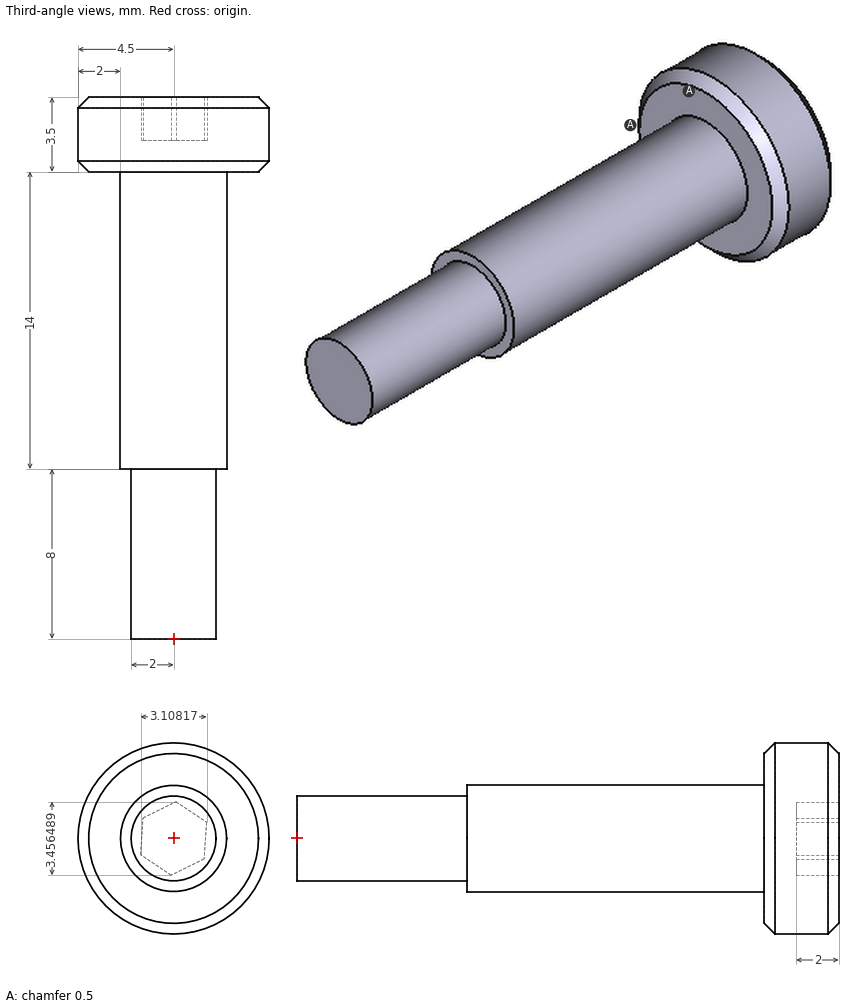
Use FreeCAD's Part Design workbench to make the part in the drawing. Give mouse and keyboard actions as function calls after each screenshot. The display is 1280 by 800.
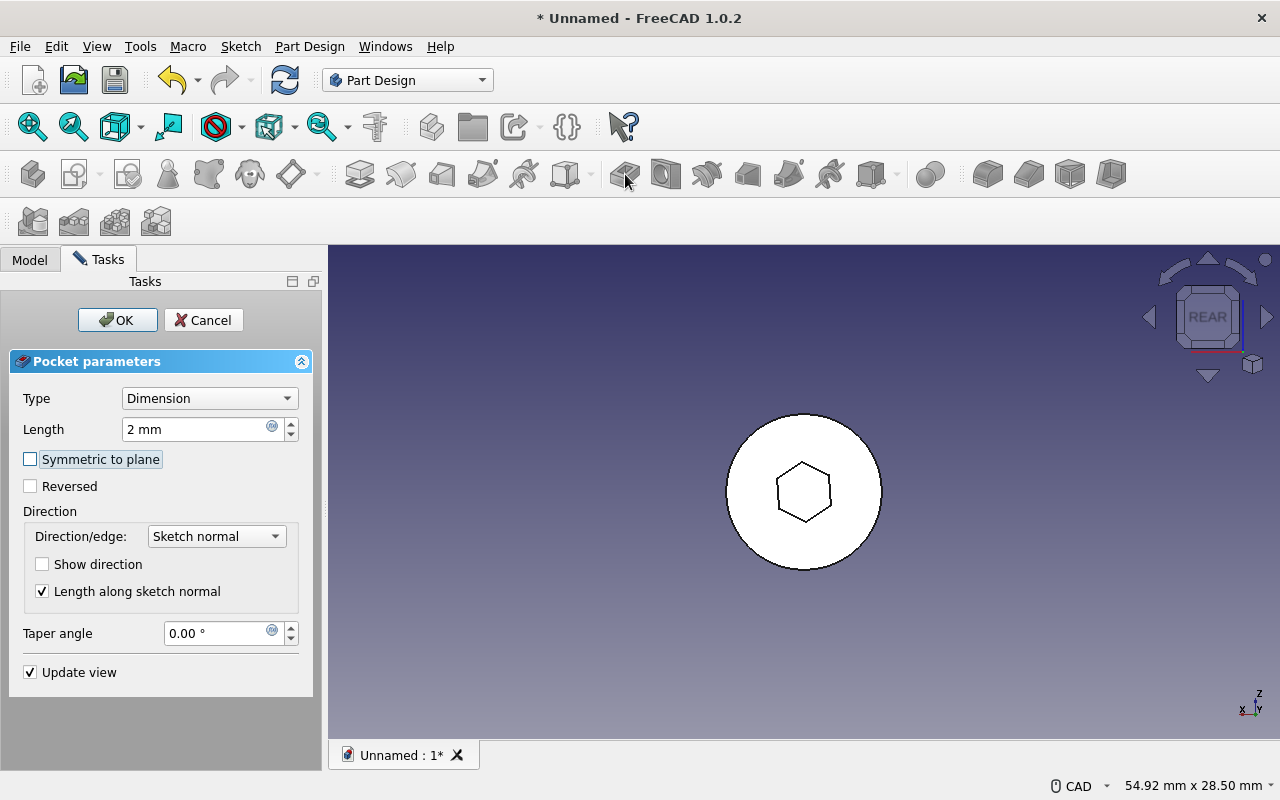
click(118, 320)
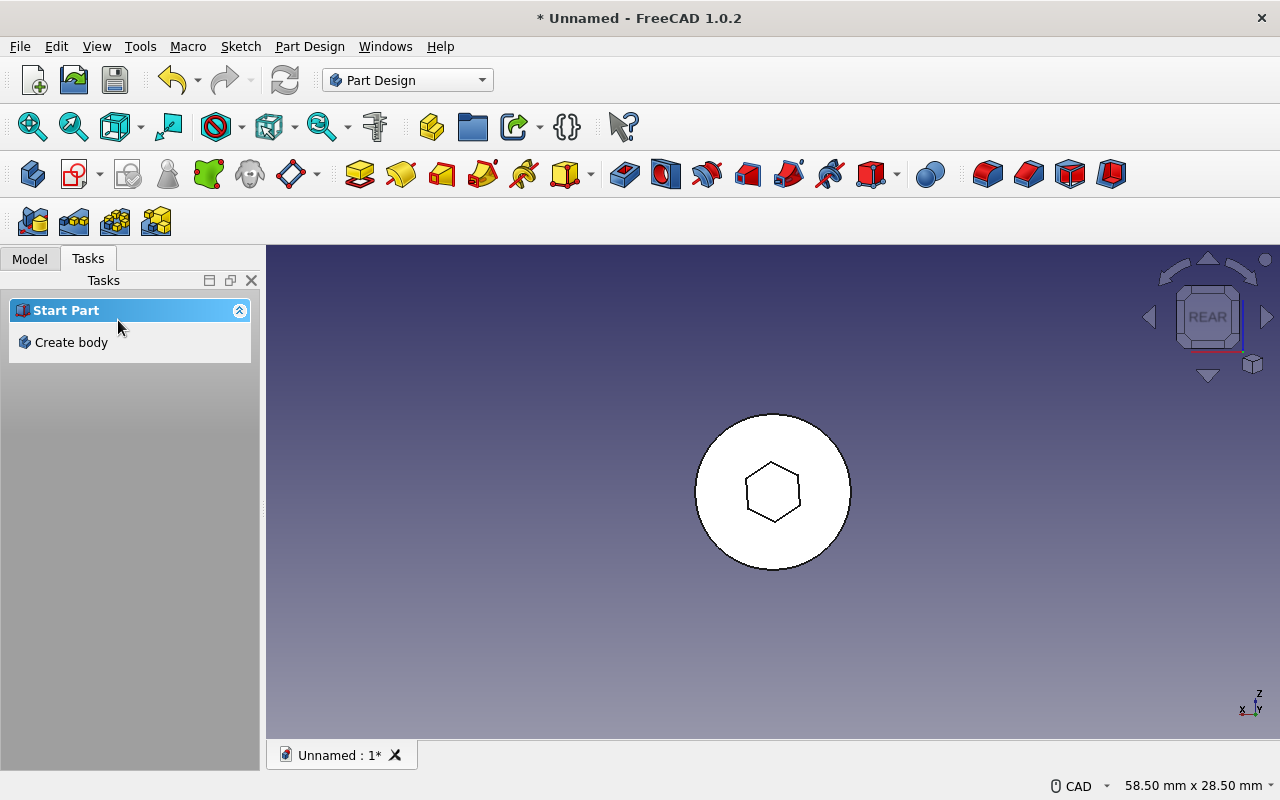
click(33, 128)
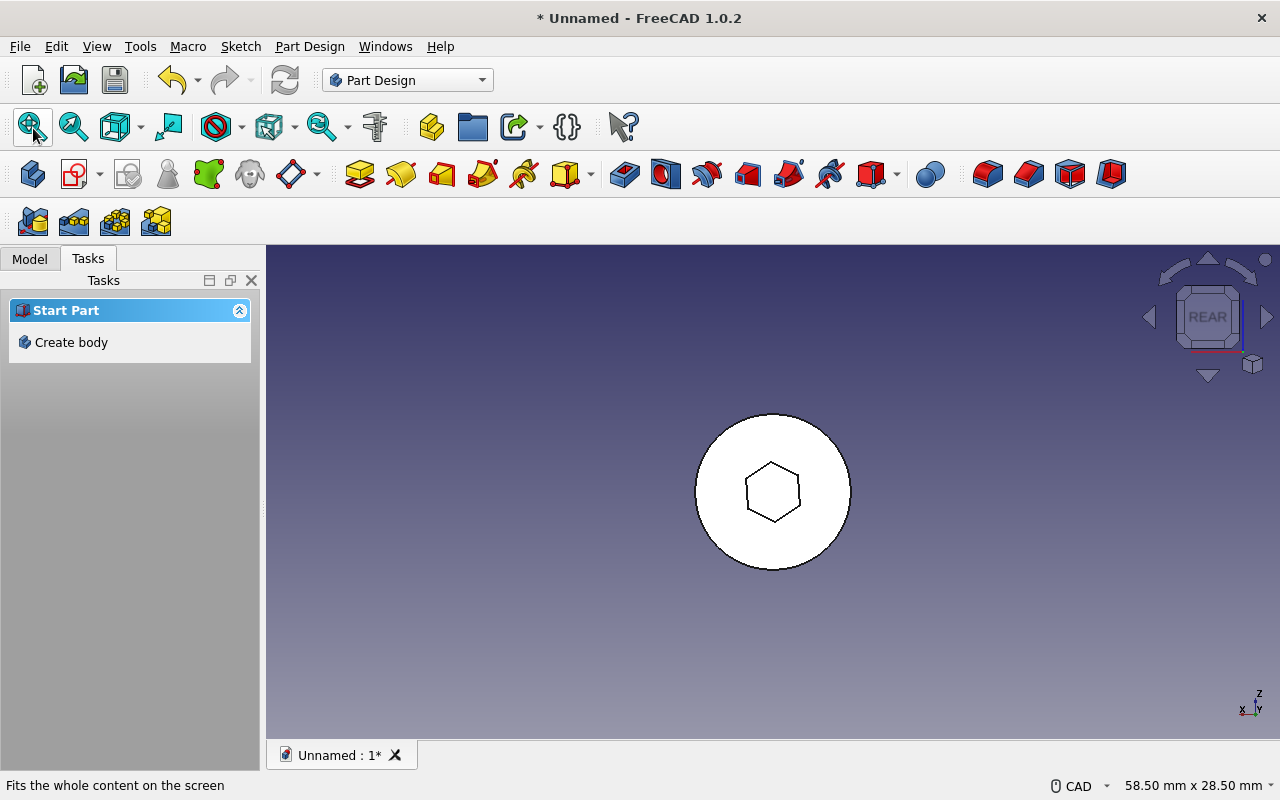
click(797, 417)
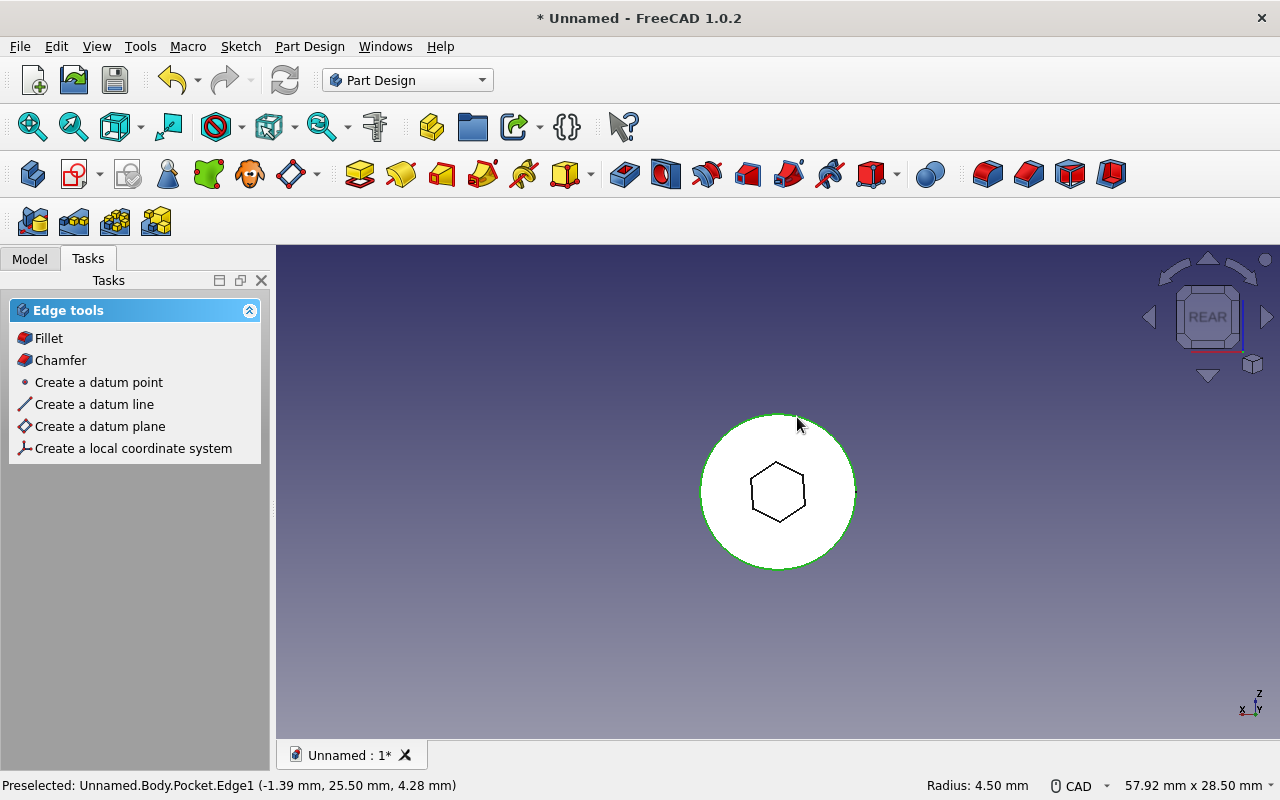
key(0)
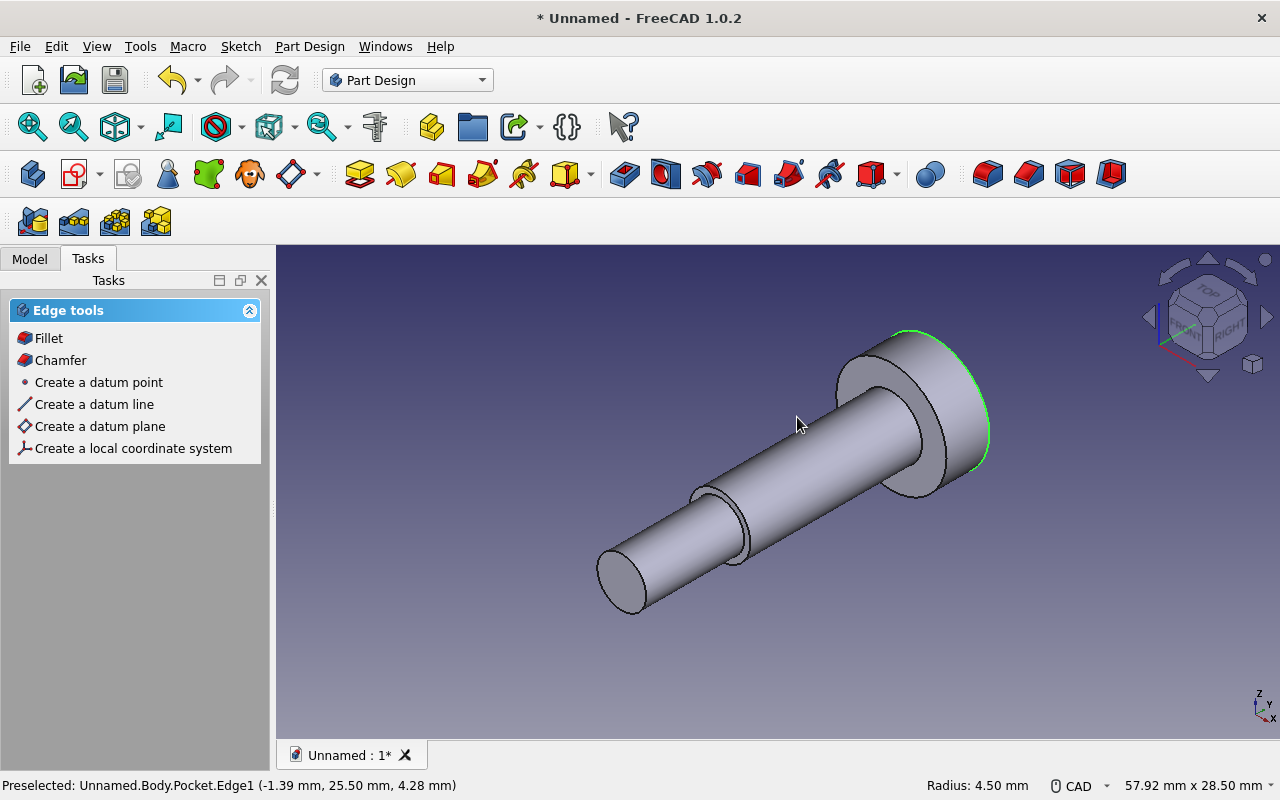
click(947, 457, ctrl)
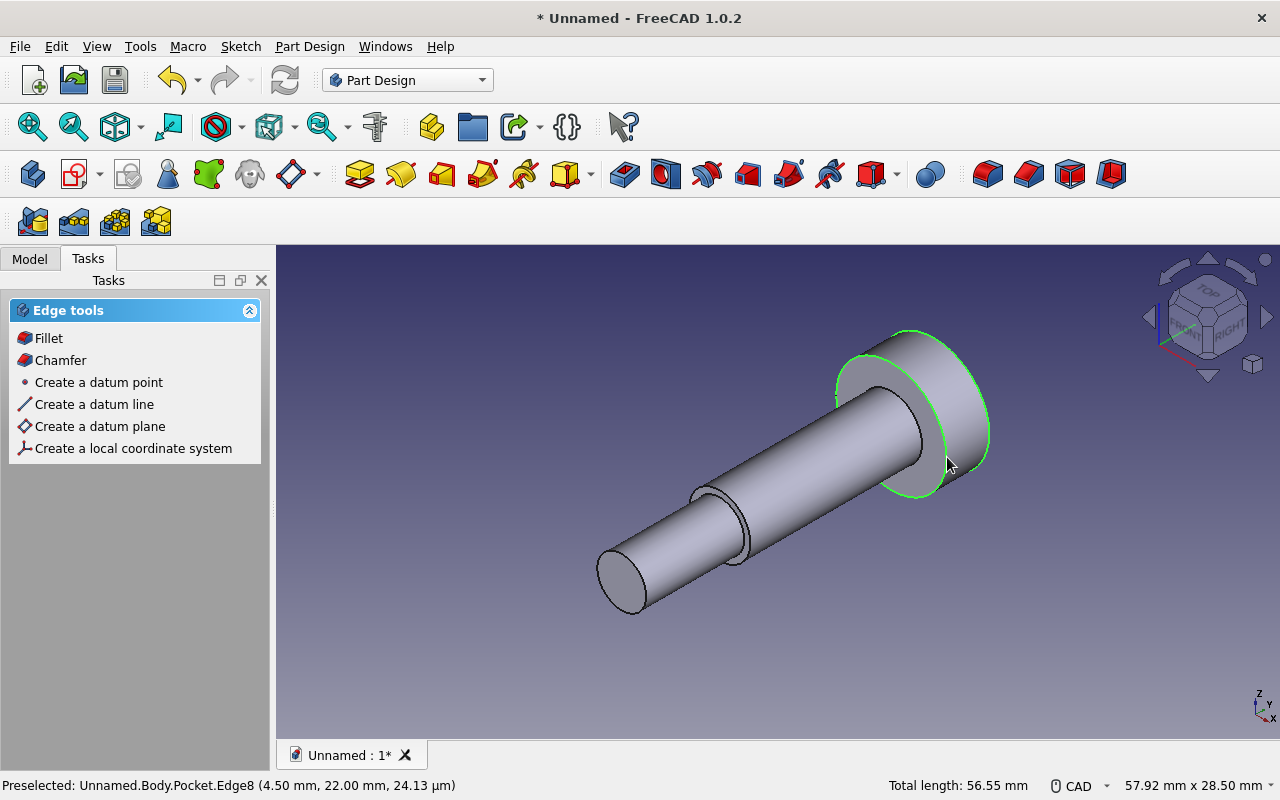
click(1029, 174)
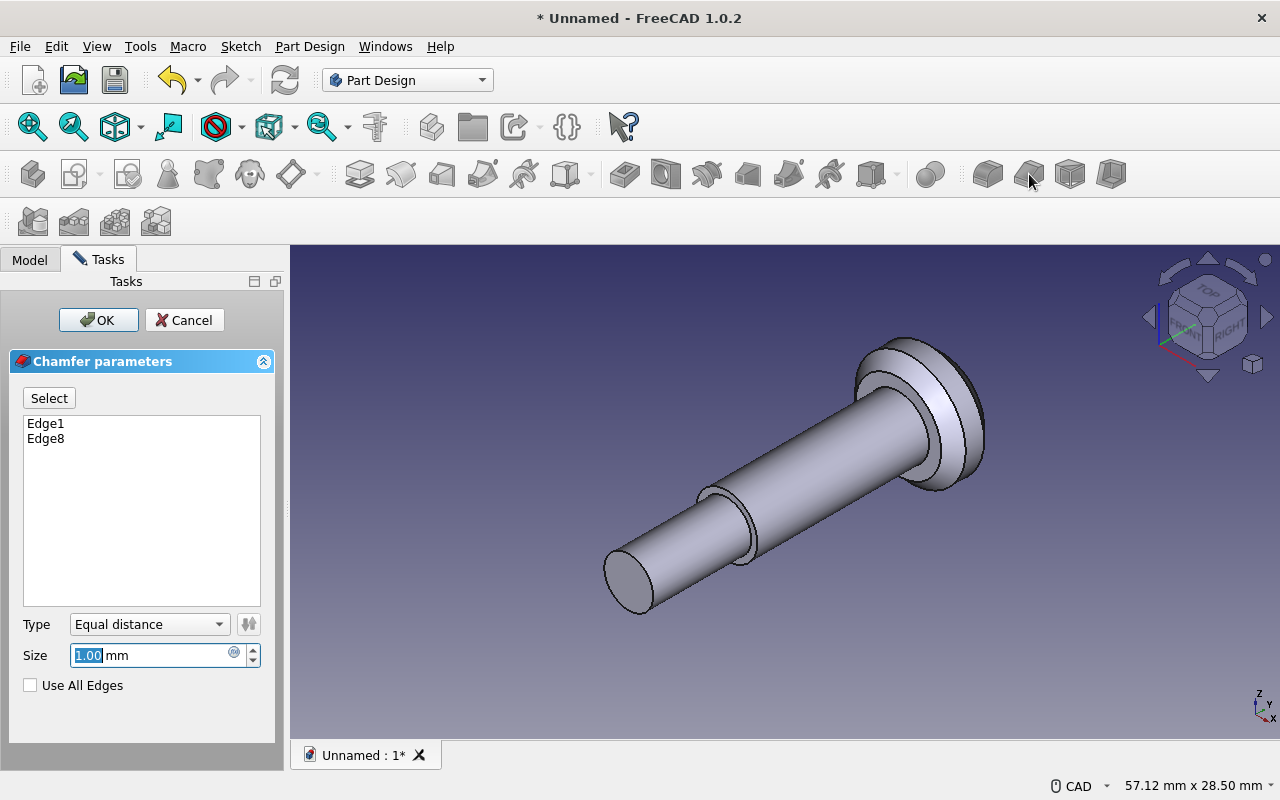
text(0.5)
key(Tab)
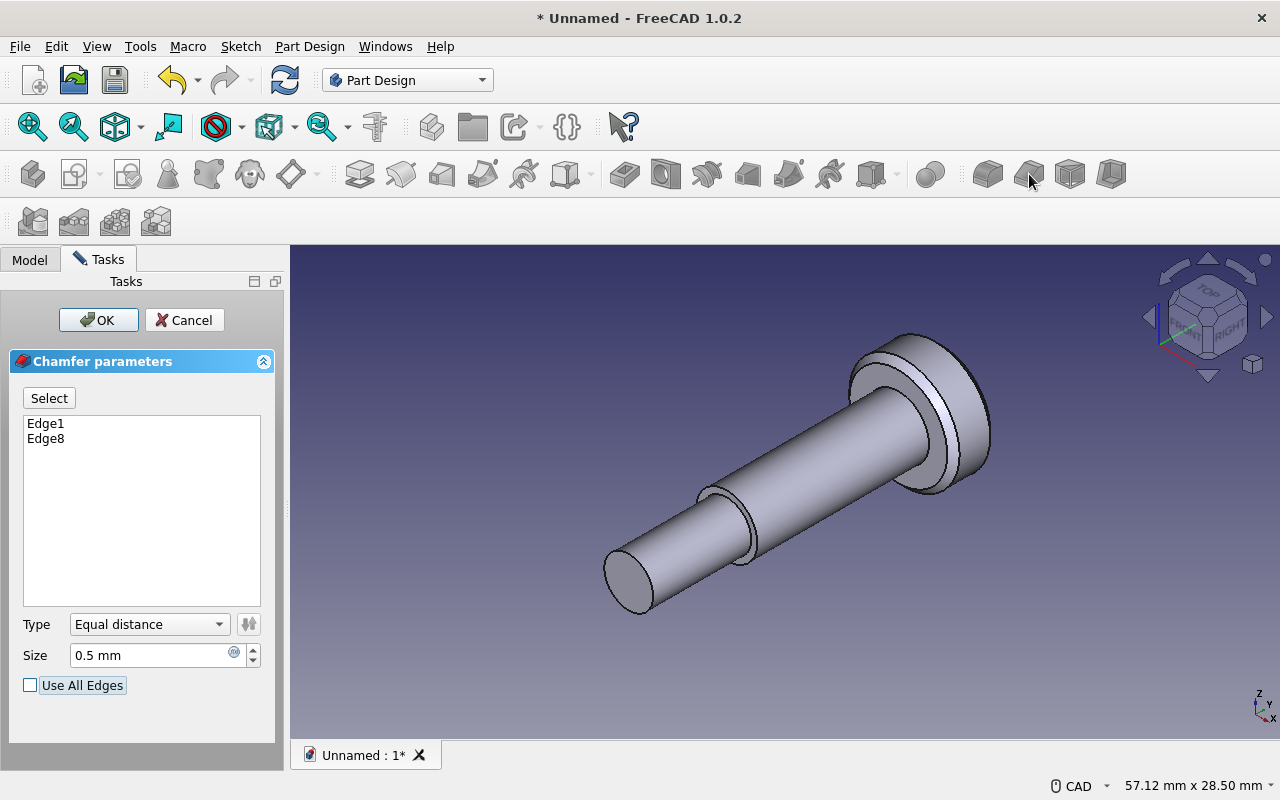
click(99, 320)